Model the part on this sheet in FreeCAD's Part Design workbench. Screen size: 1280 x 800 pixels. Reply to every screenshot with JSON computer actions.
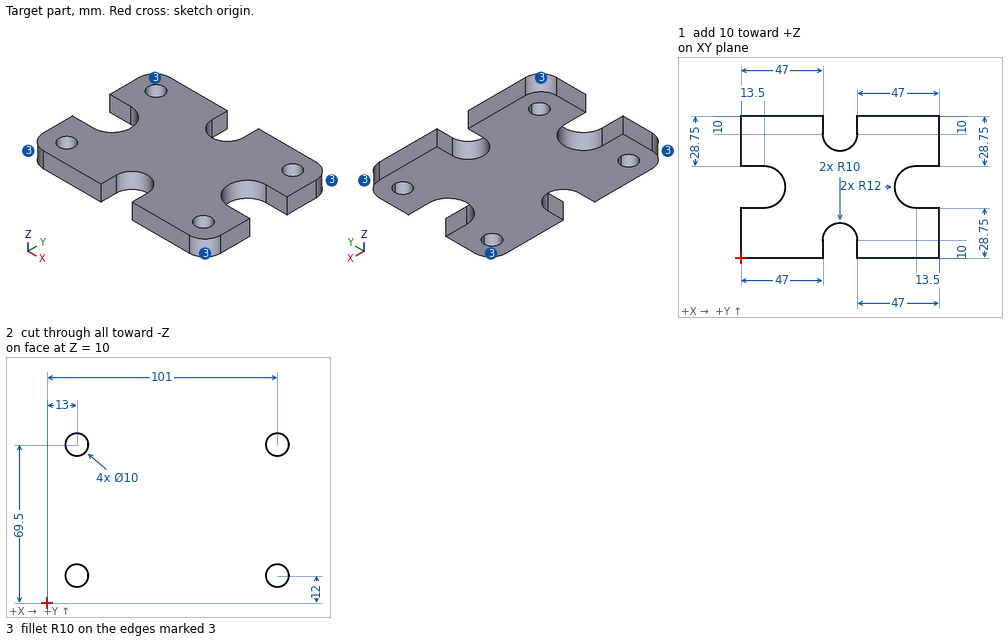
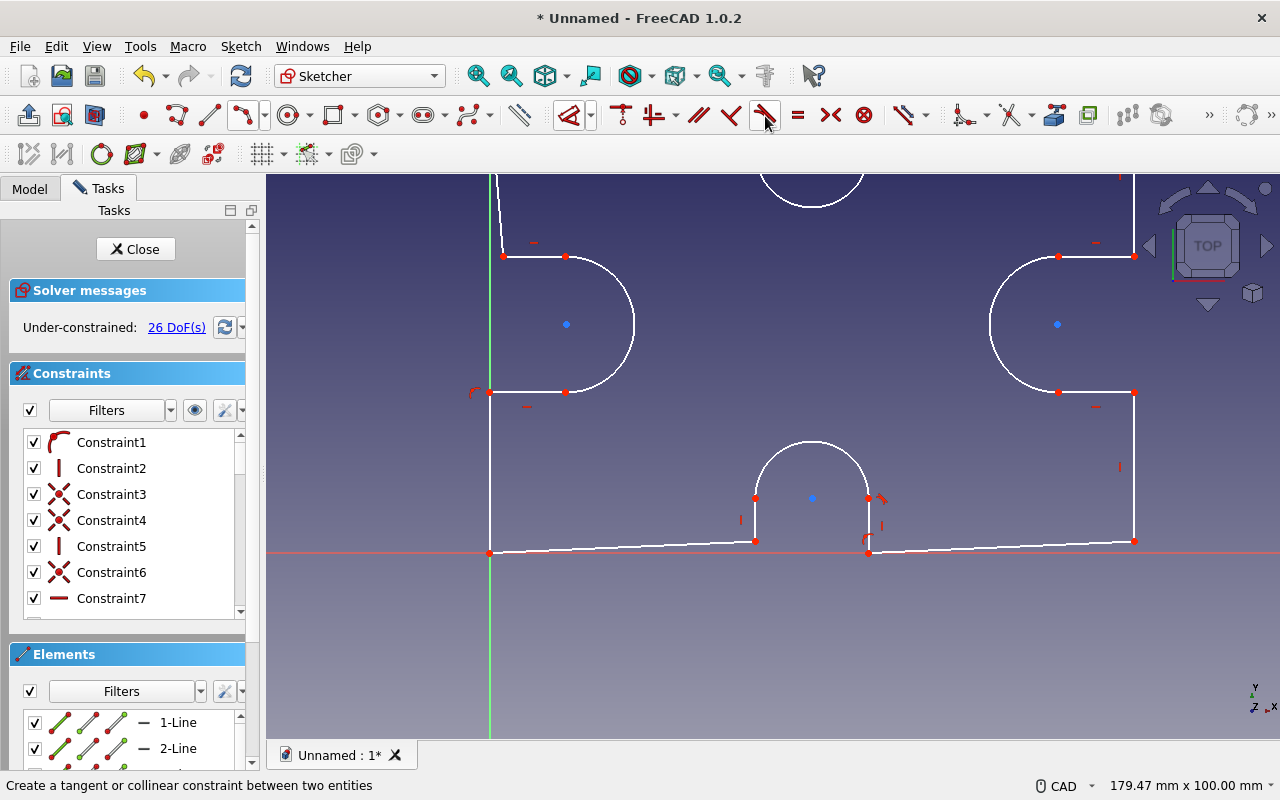
{"action": "left_click", "coordinate": [1111, 392]}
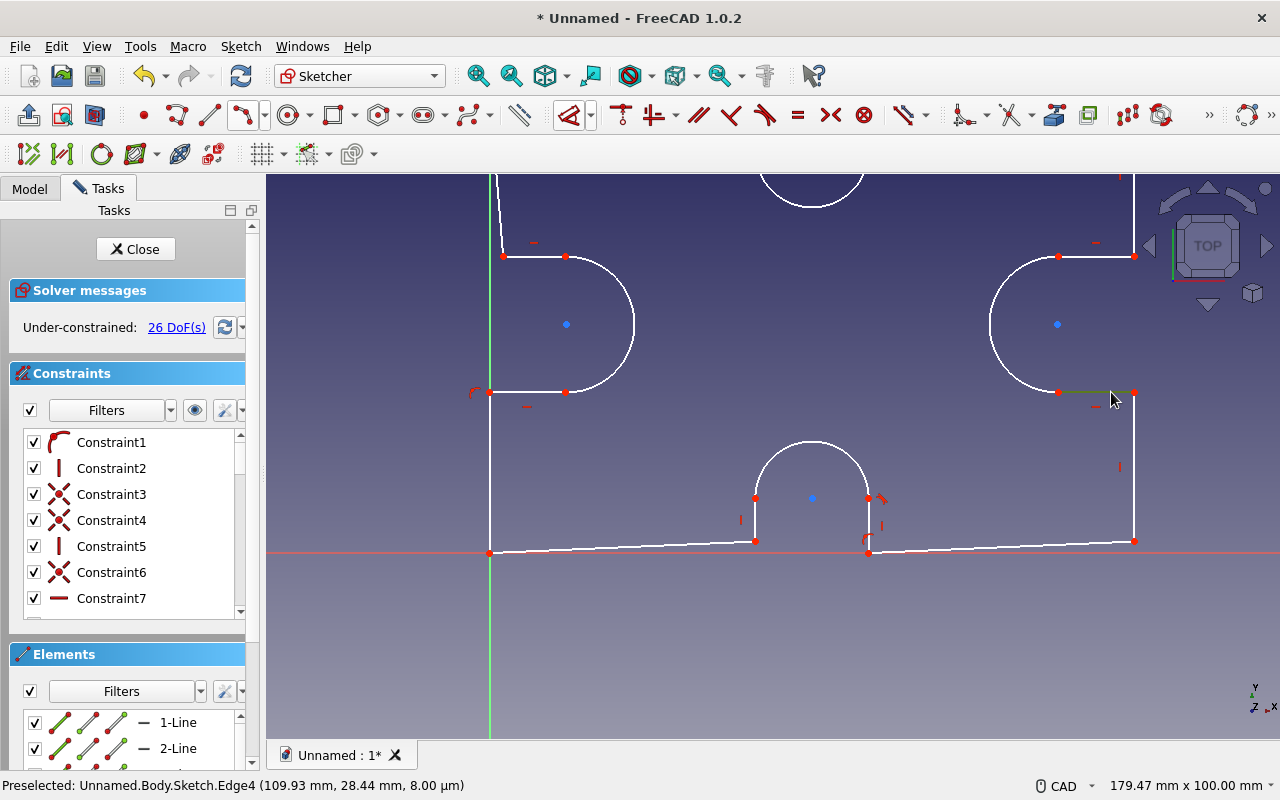
{"action": "left_click", "coordinate": [1003, 284]}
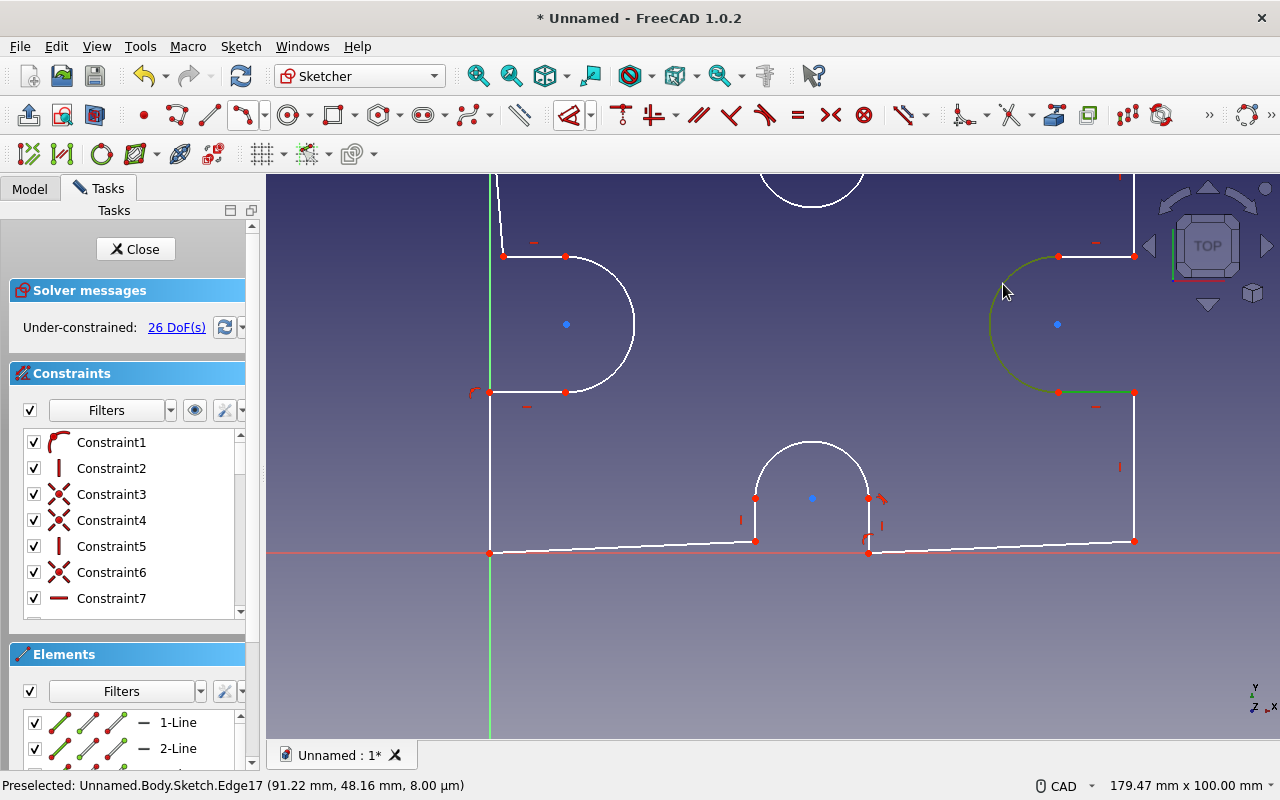
{"action": "left_click", "coordinate": [765, 116]}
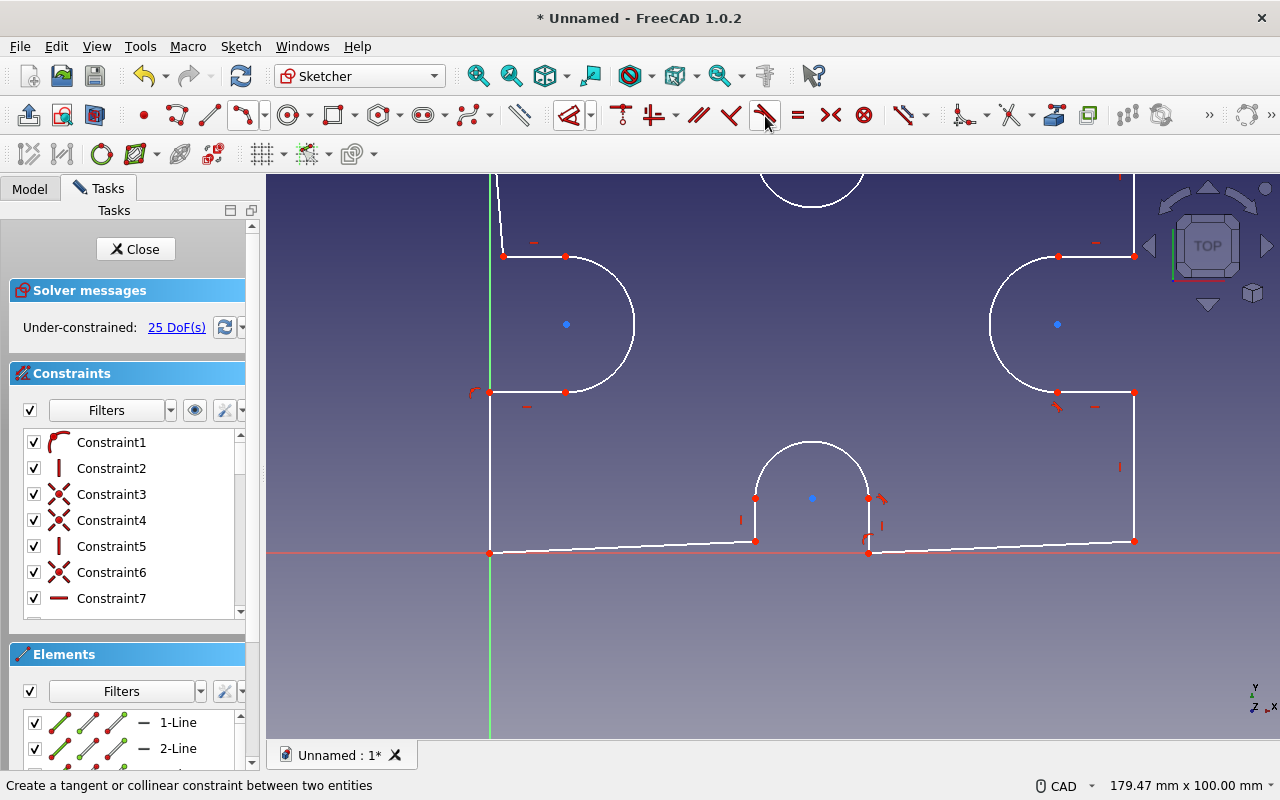
{"action": "left_click", "coordinate": [1081, 257]}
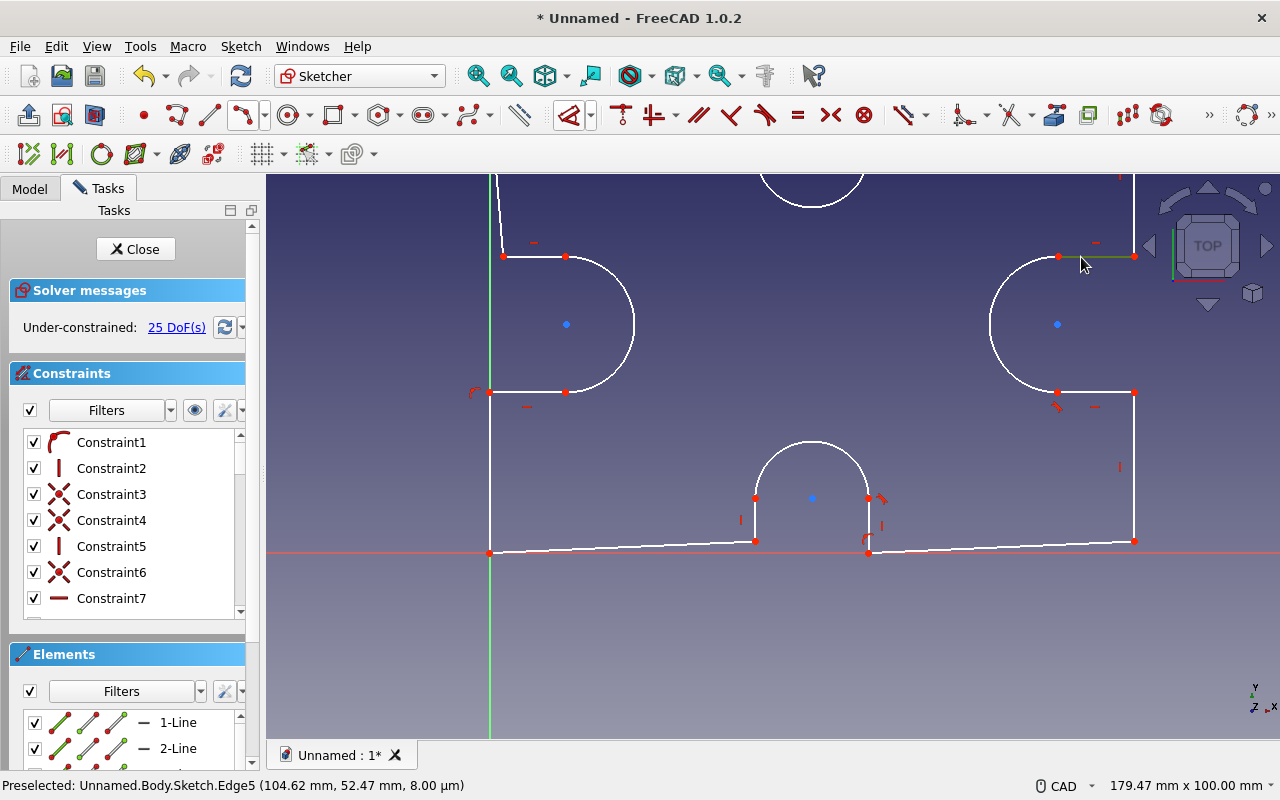
{"action": "left_click", "coordinate": [1003, 284]}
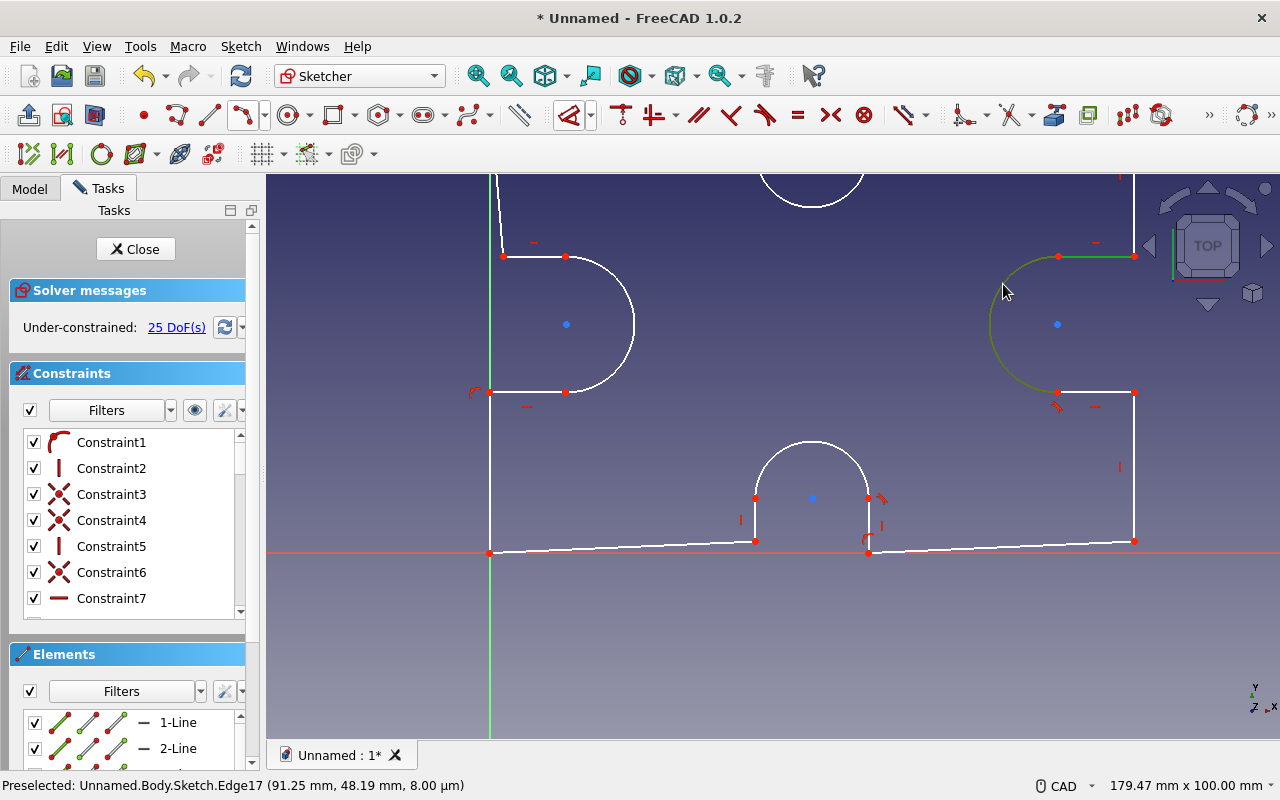
{"action": "left_click", "coordinate": [765, 116]}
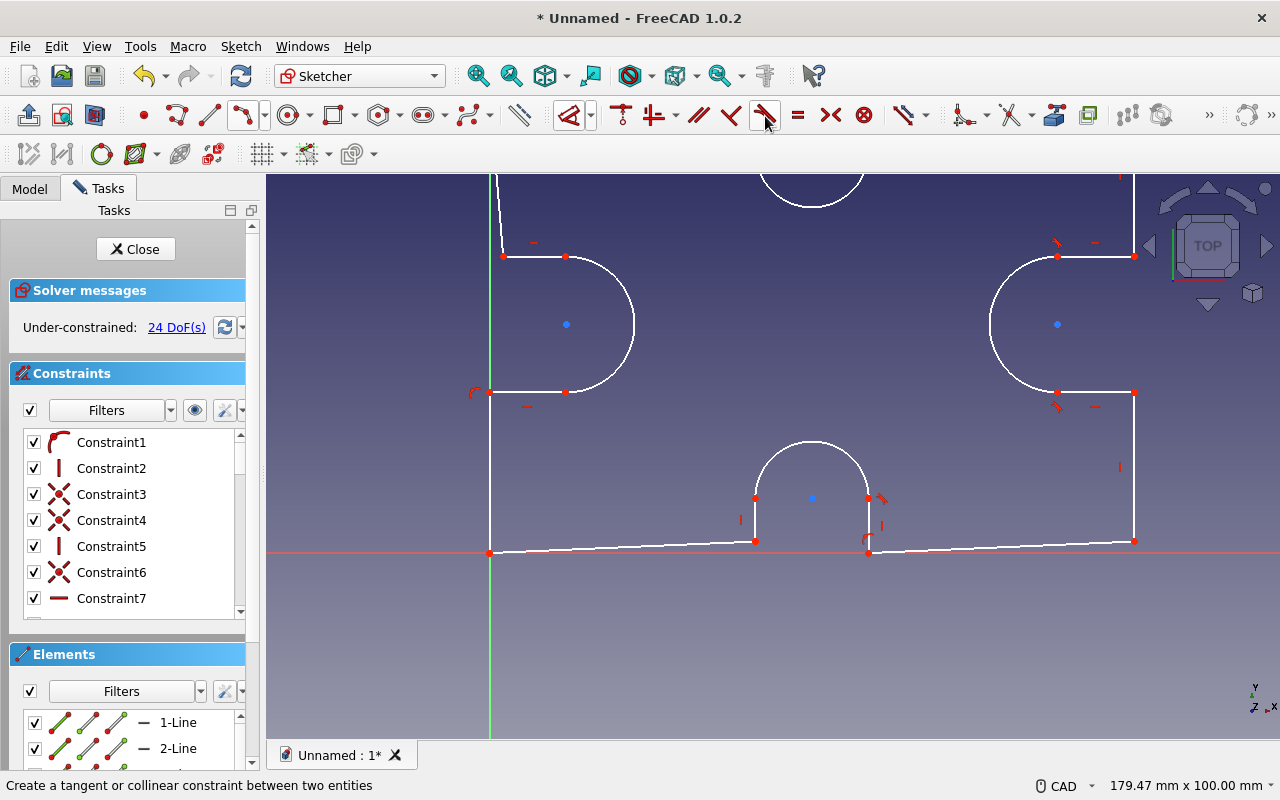
{"action": "scroll", "coordinate": [486, 711], "scroll_direction": "down", "scroll_amount": 2}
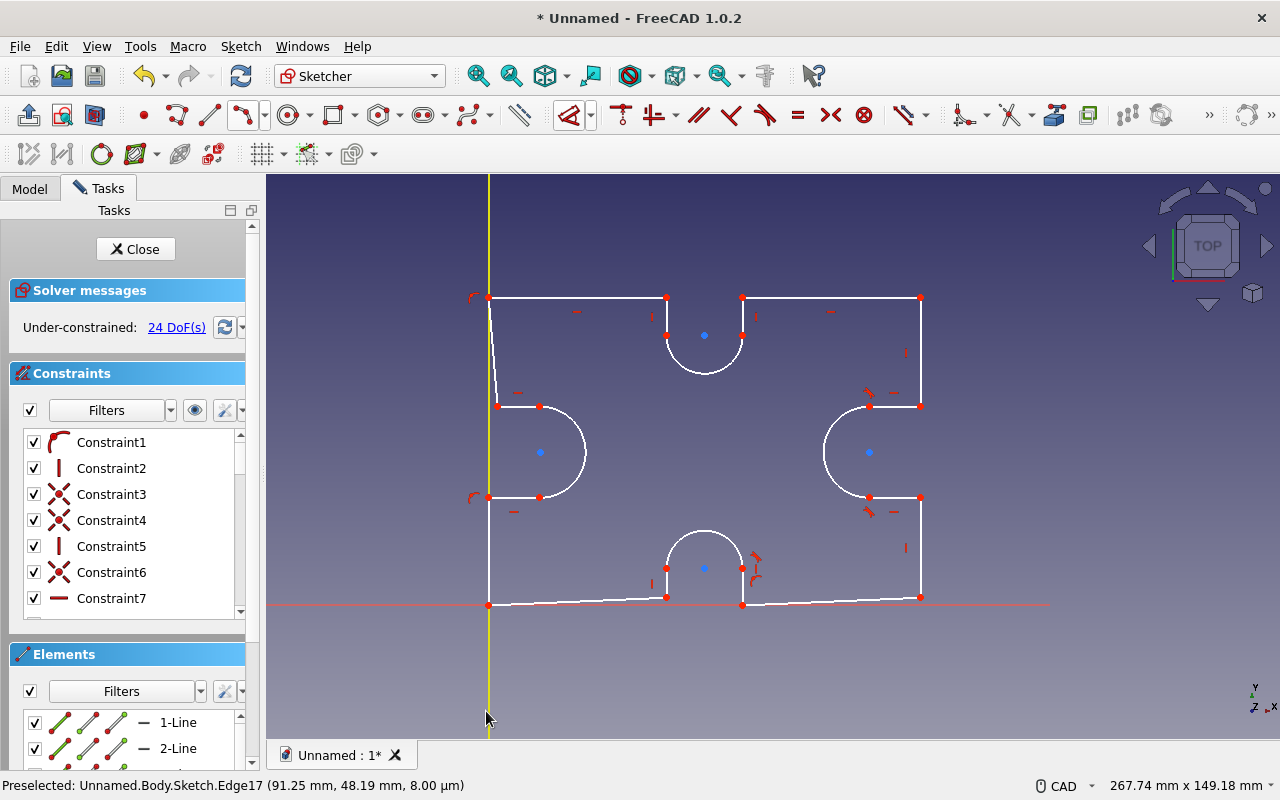
{"action": "left_click", "coordinate": [743, 309]}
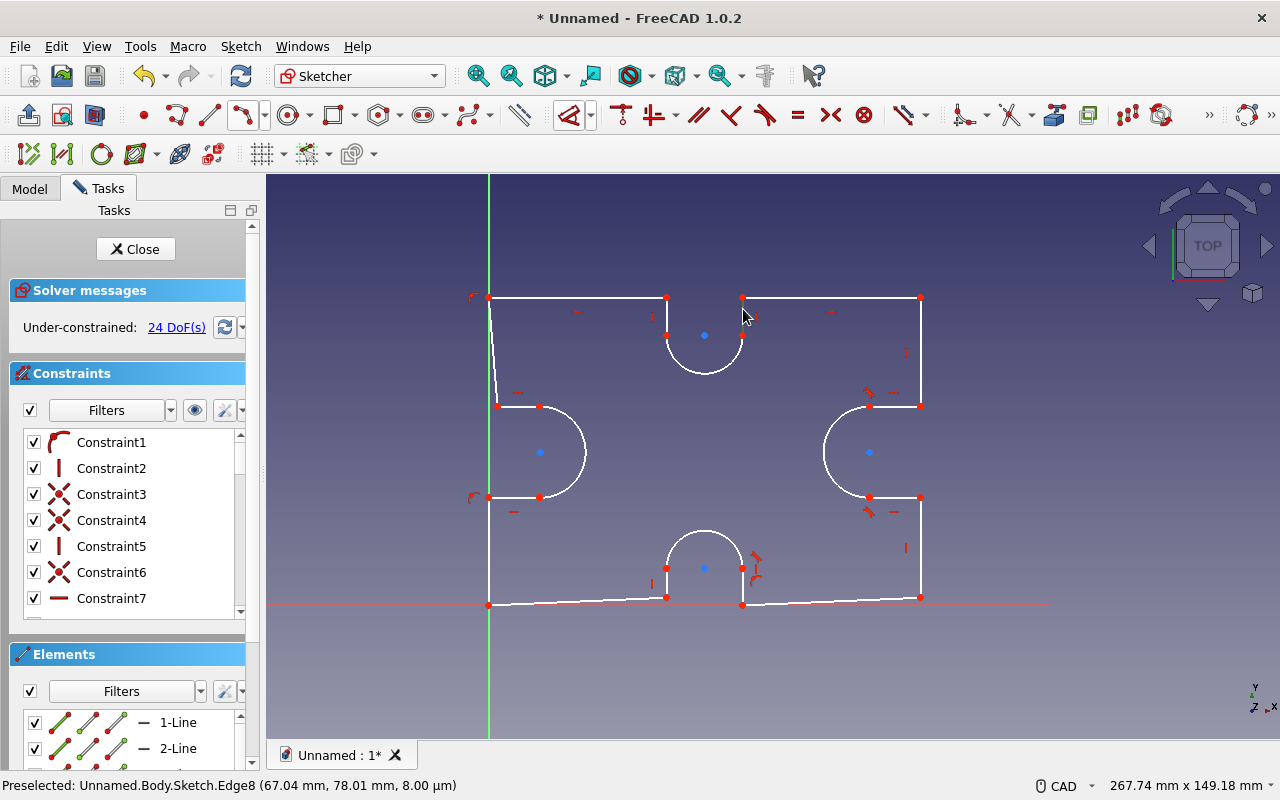
{"action": "left_click", "coordinate": [682, 366]}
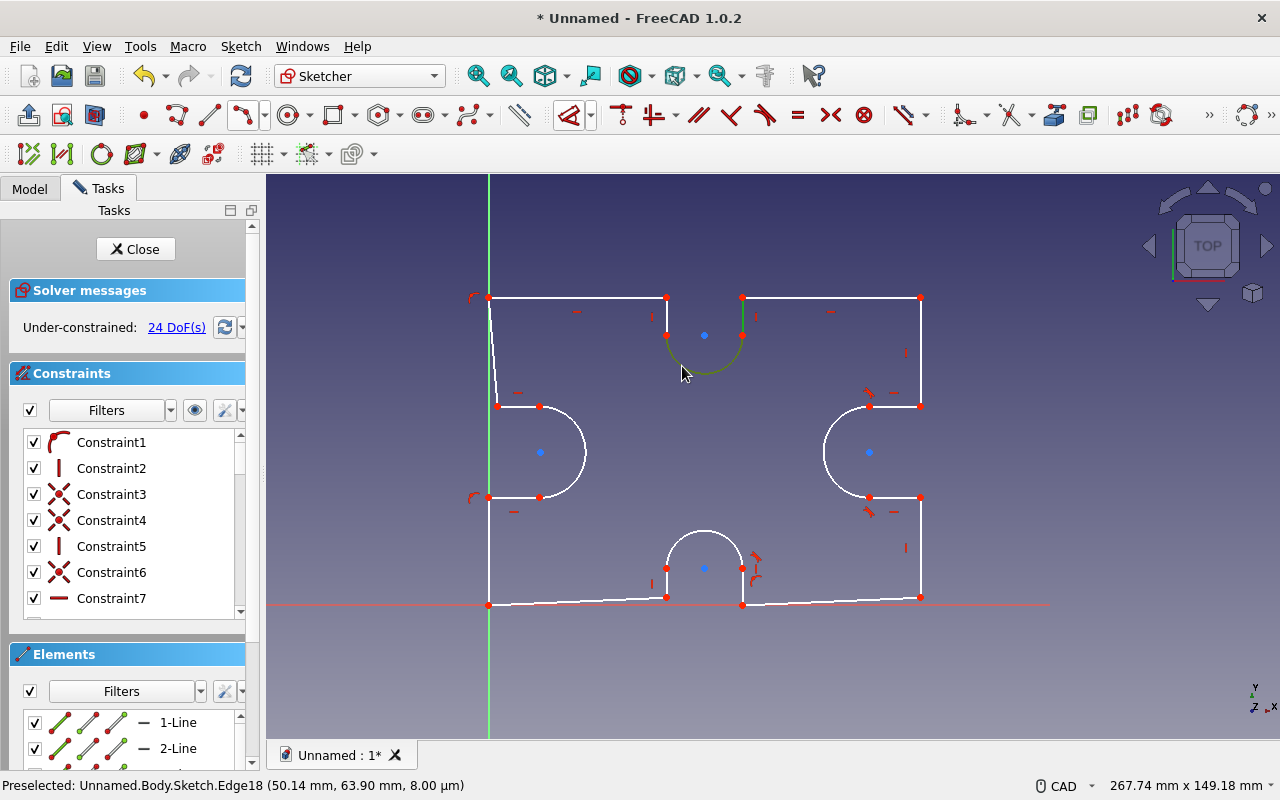
{"action": "left_click", "coordinate": [765, 116]}